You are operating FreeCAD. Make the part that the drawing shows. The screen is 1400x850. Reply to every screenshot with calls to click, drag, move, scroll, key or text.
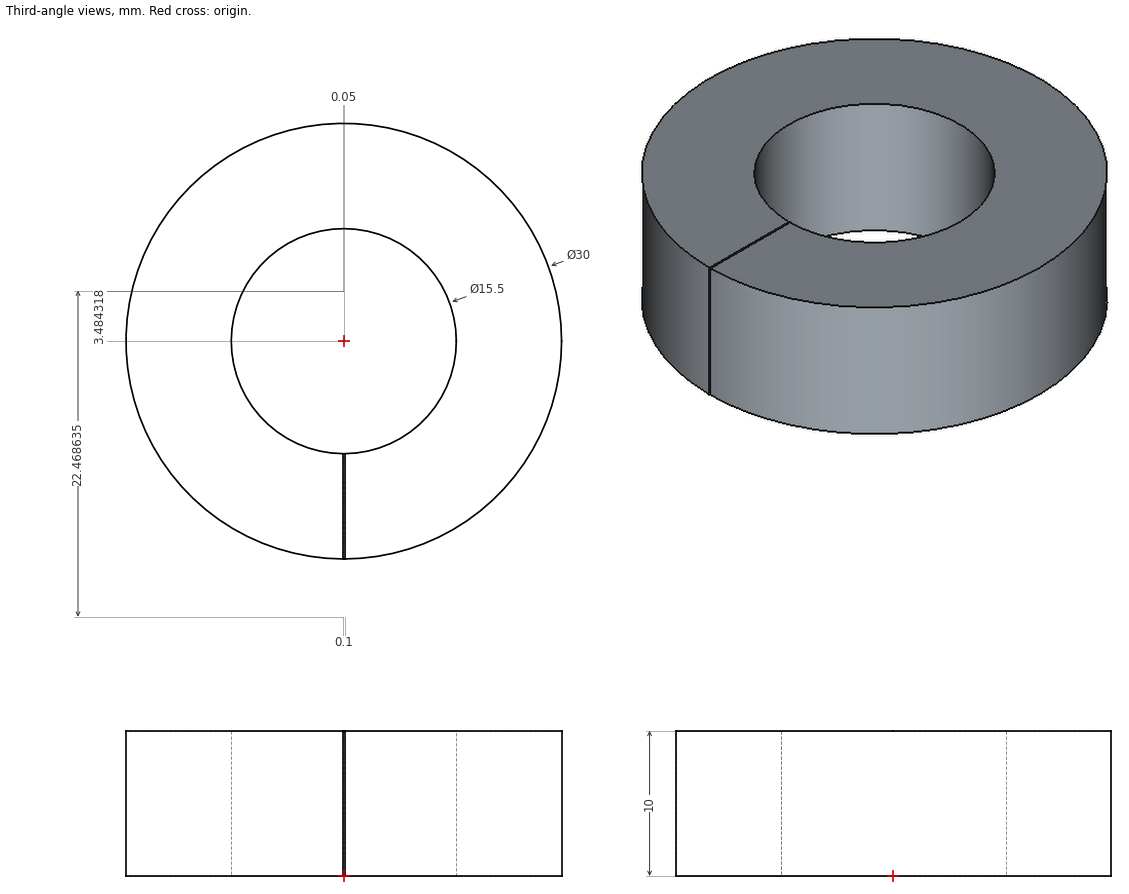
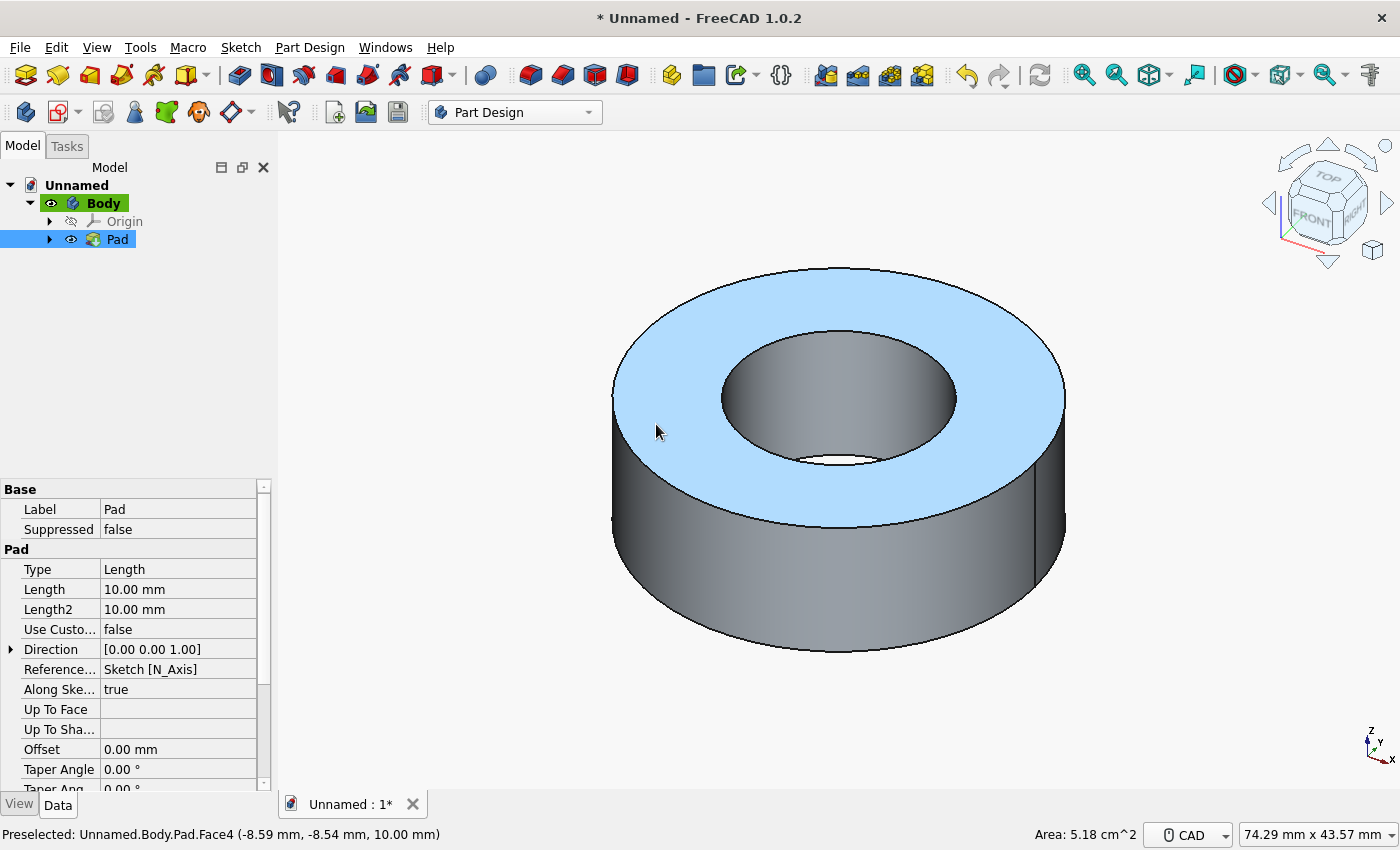
click(58, 112)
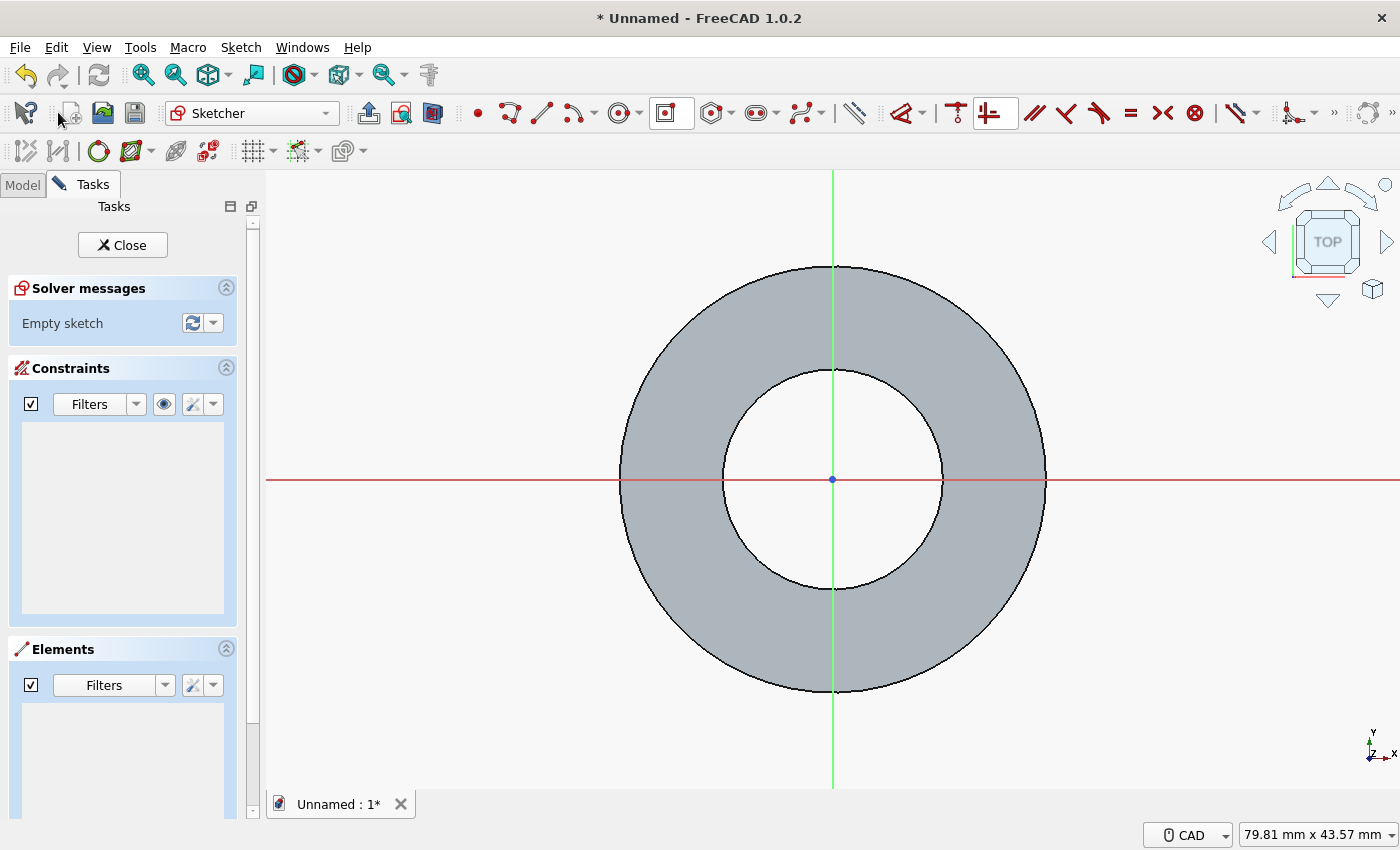
scroll(456, 198, down, 1)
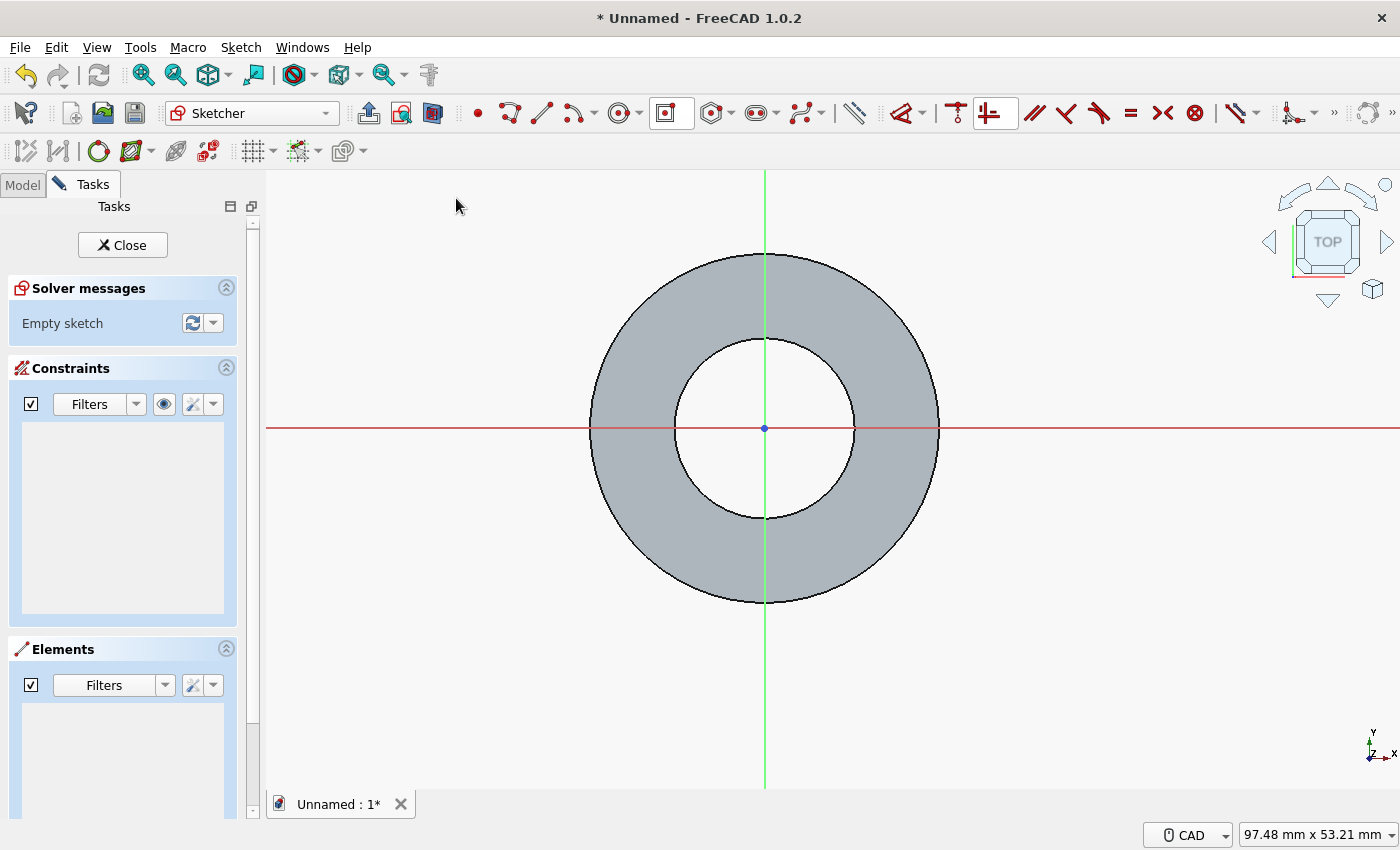
scroll(765, 598, up, 2)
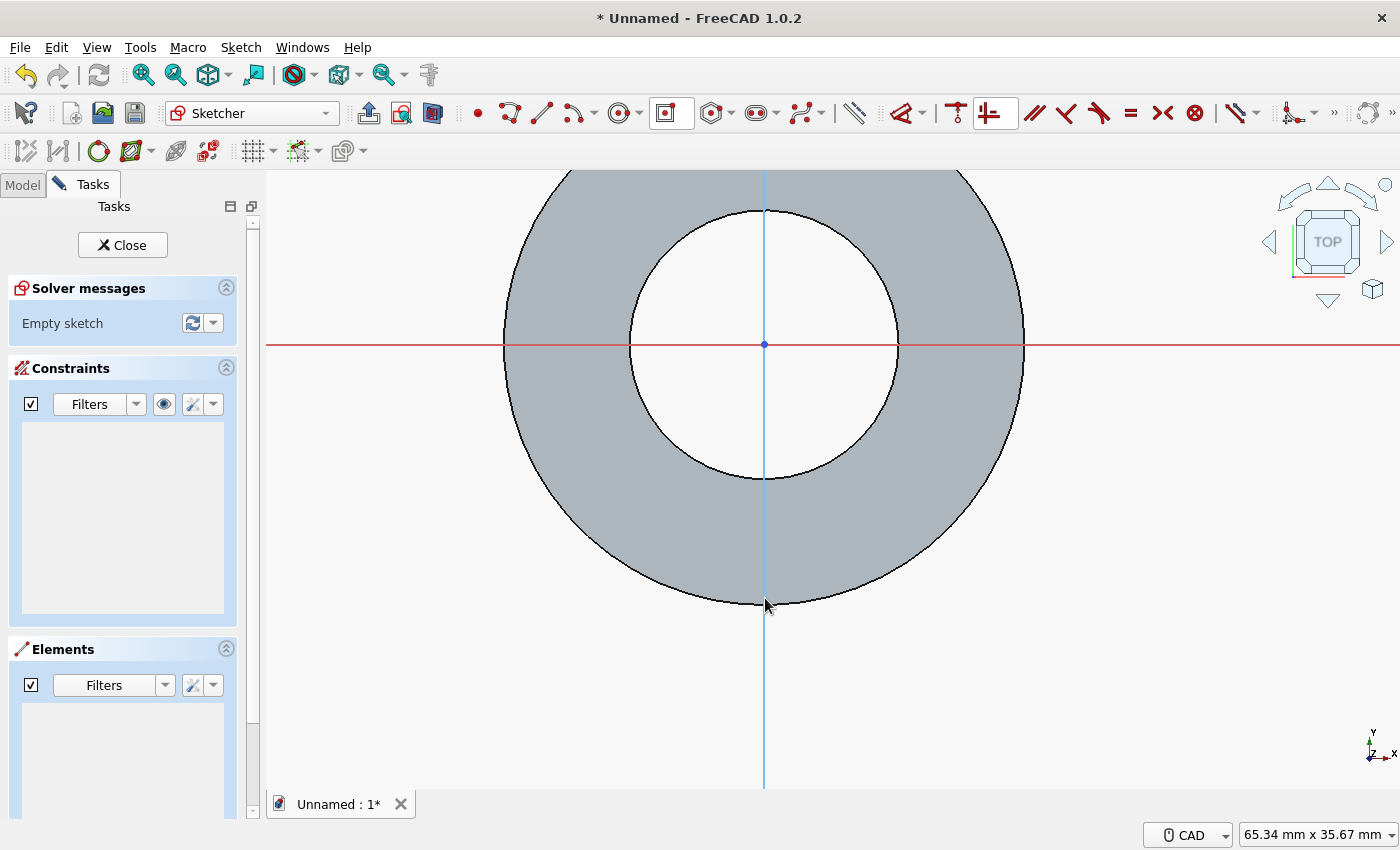
key(g)
key(r)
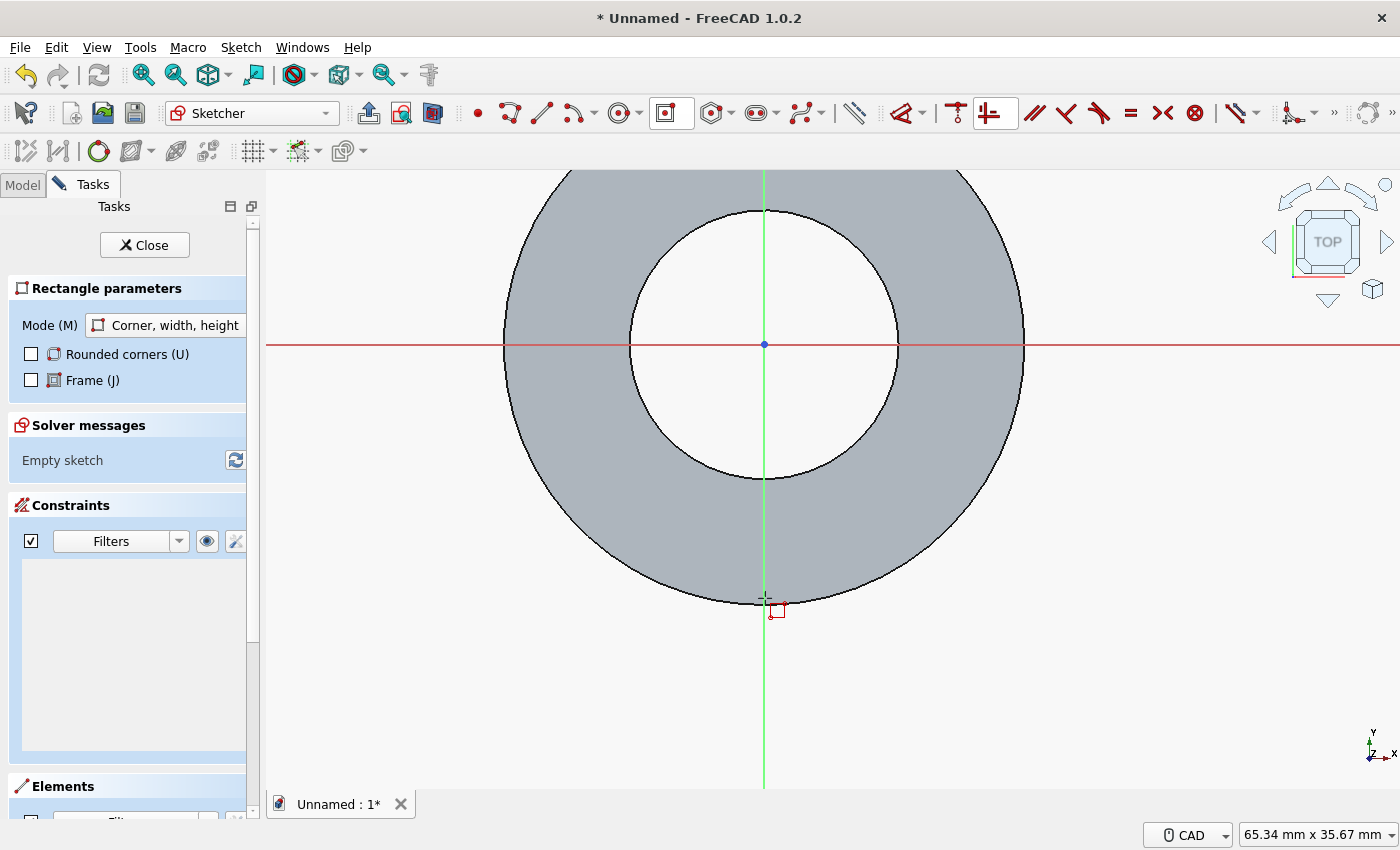
scroll(763, 284, up, 15)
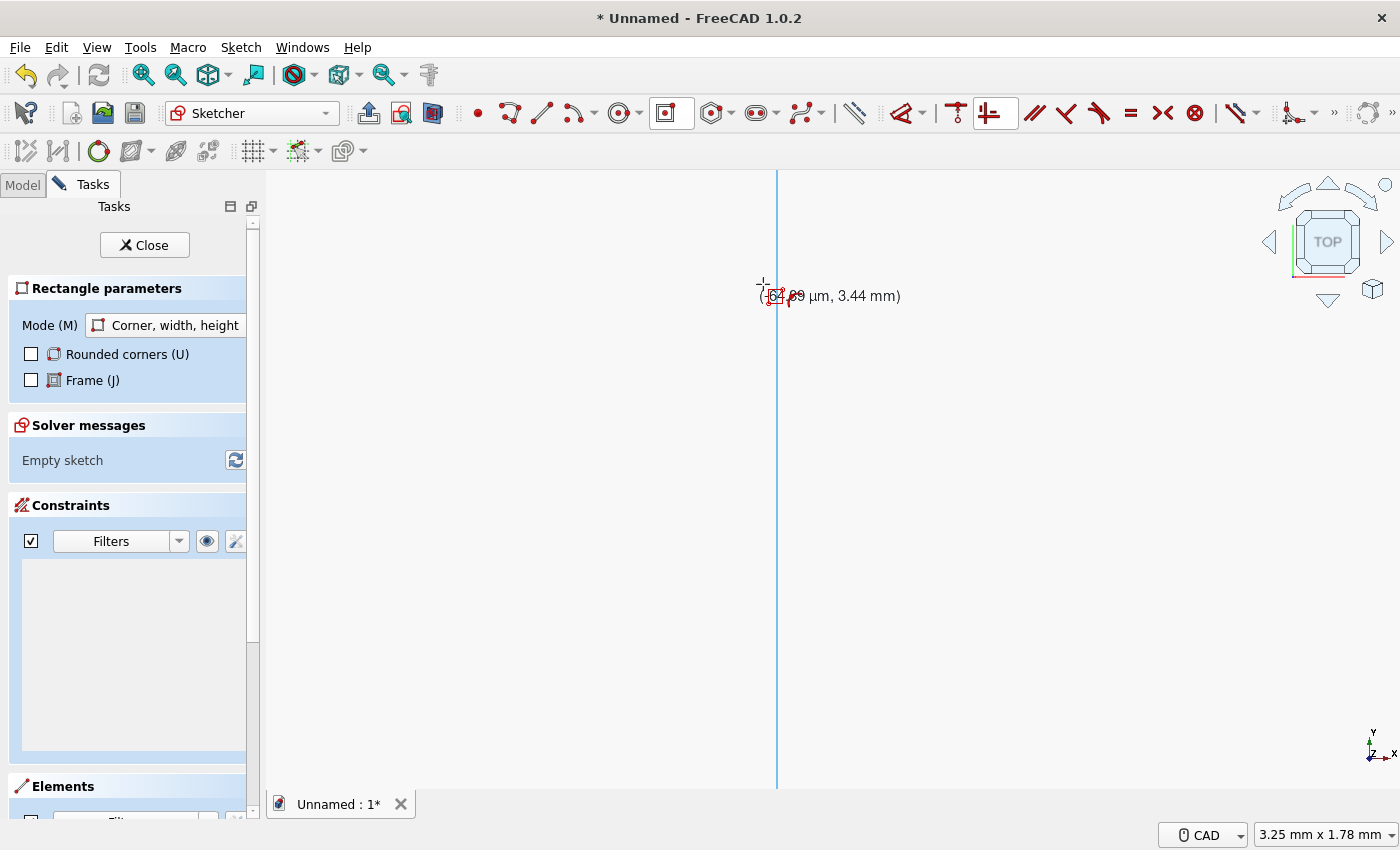
click(760, 286)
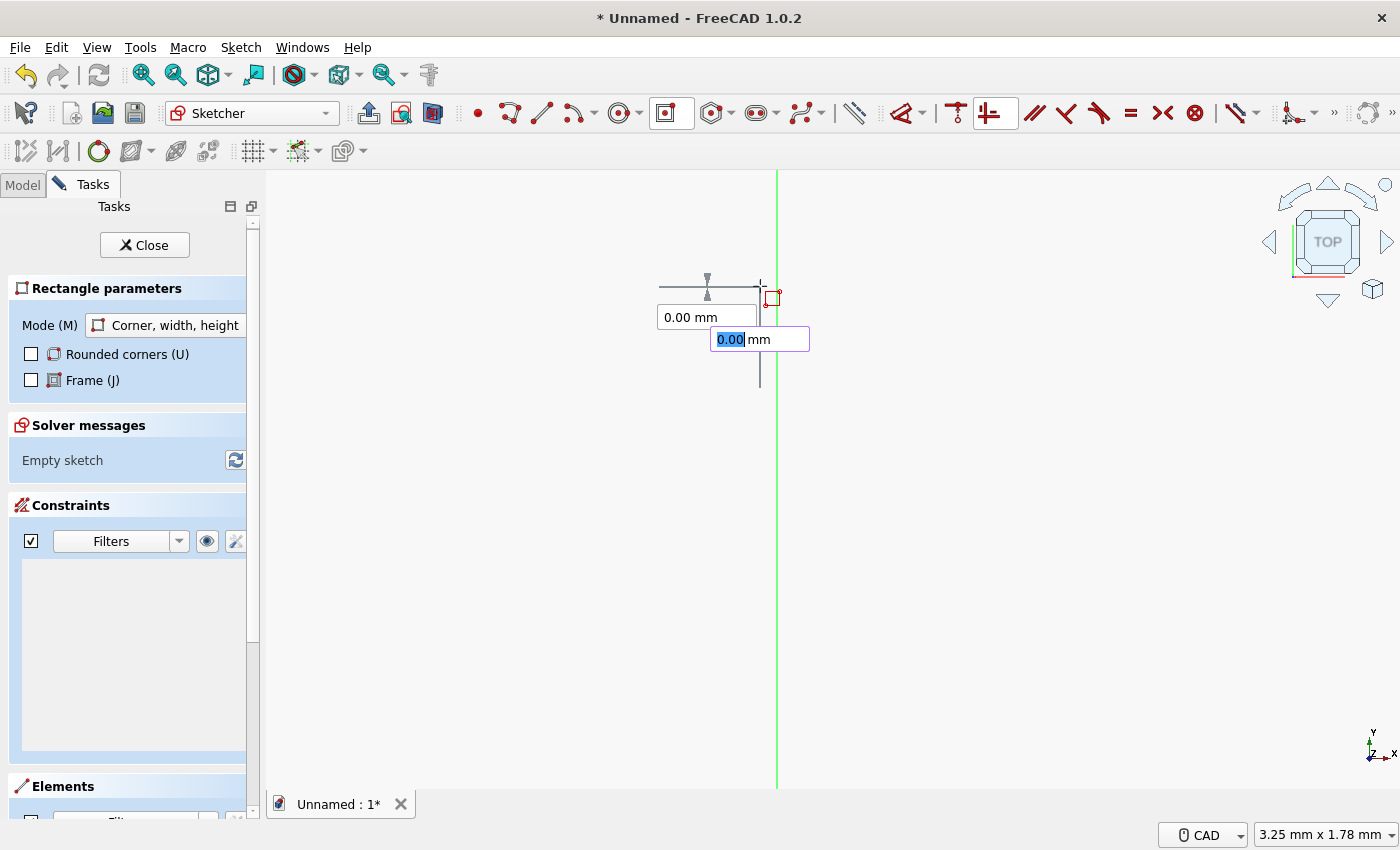
scroll(764, 284, down, 15)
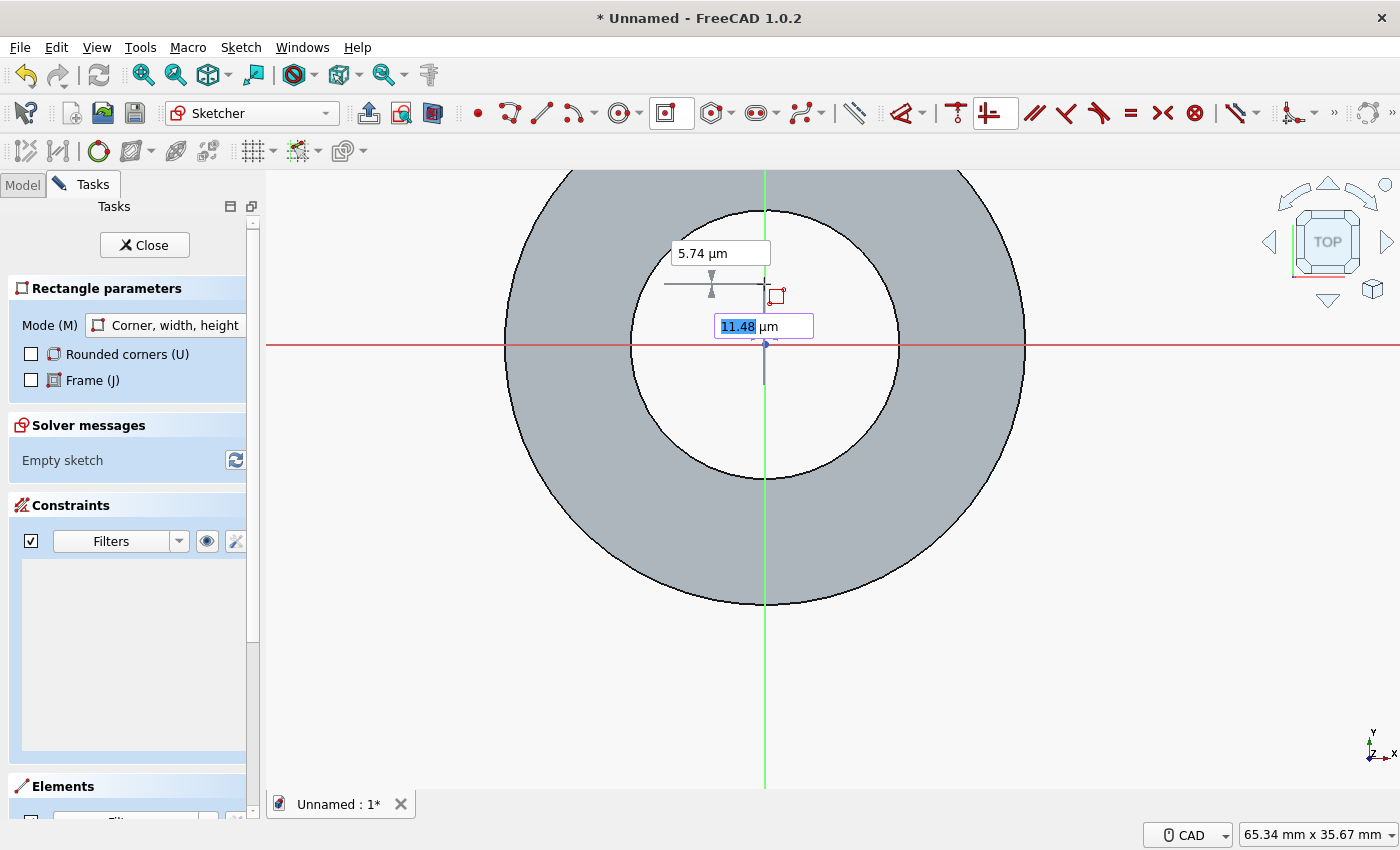
scroll(766, 674, up, 15)